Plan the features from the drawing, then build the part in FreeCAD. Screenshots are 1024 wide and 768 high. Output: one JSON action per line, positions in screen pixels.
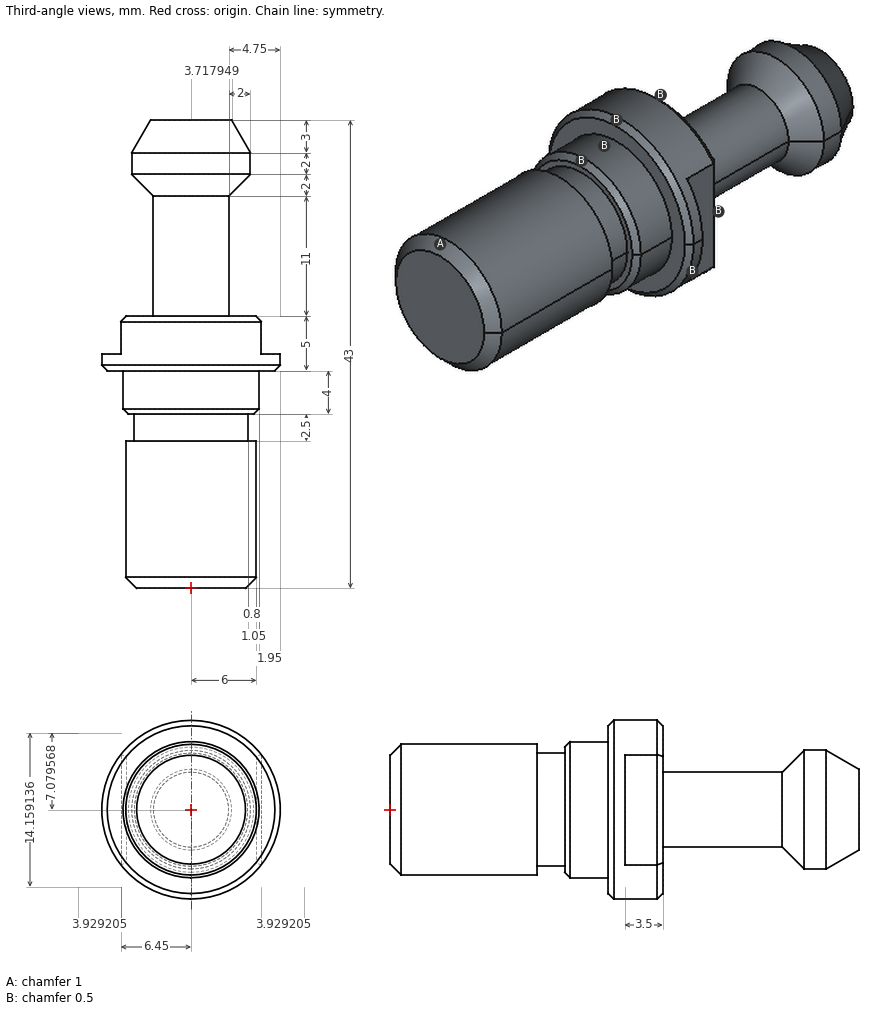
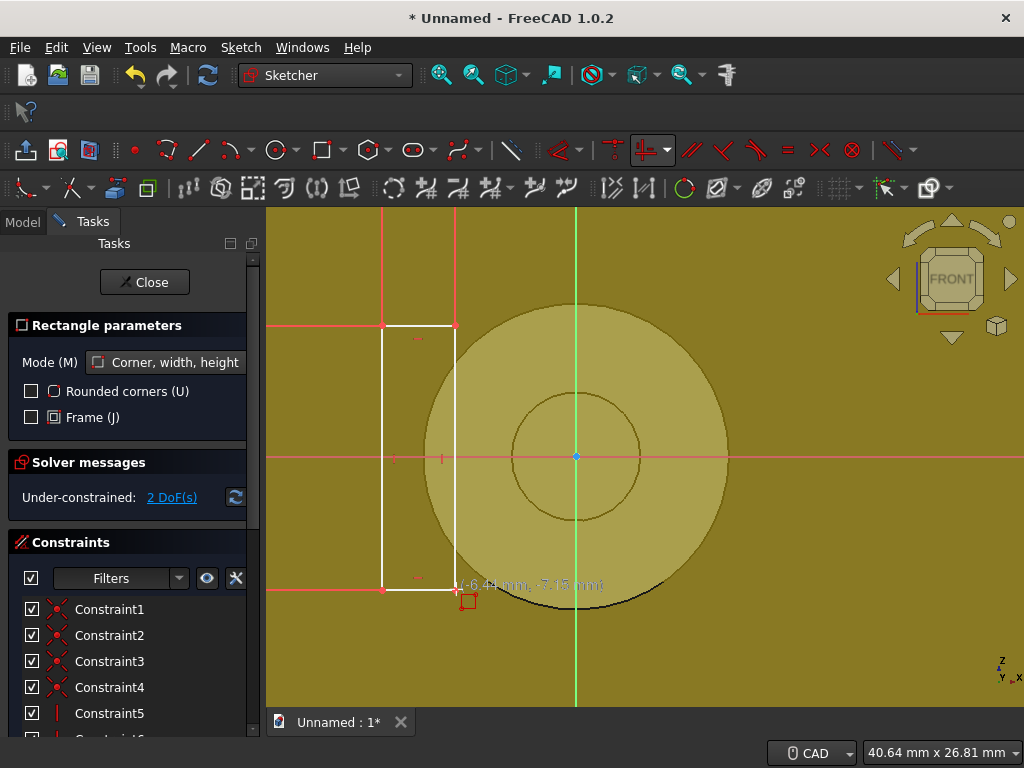
{"action": "left_click", "coordinate": [696, 325]}
{"action": "mouse_move", "coordinate": [770, 589]}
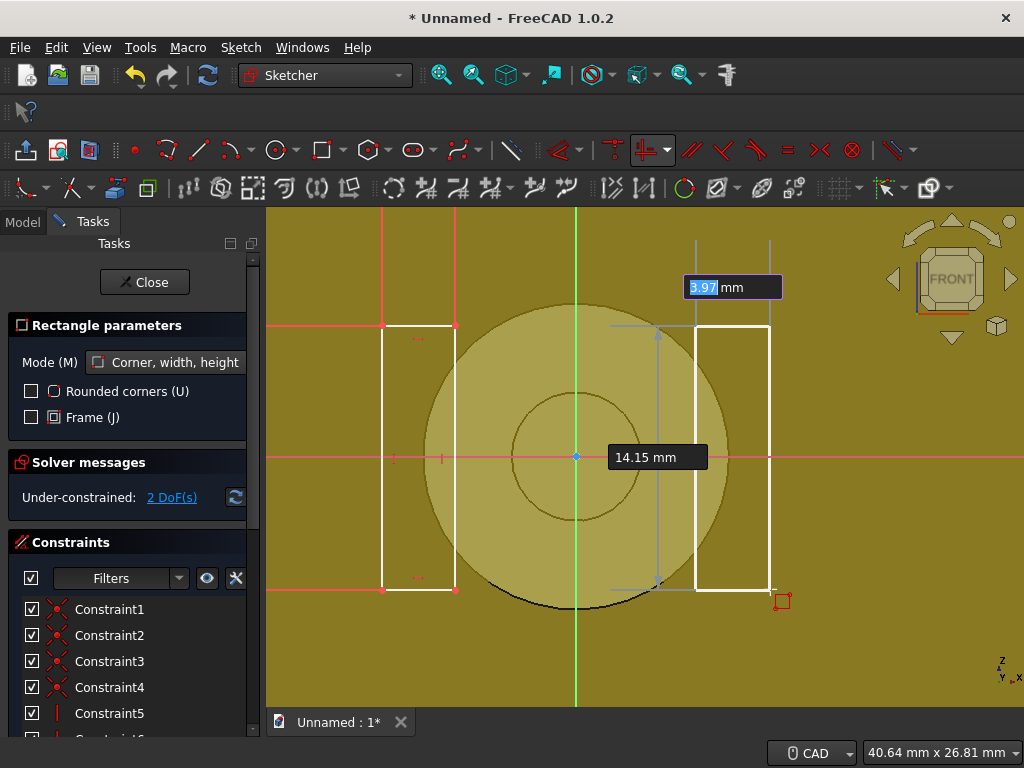
{"action": "type", "text": "3.929205"}
{"action": "key", "text": "Tab"}
{"action": "type", "text": "14.159136"}
{"action": "key", "text": "Return"}
{"action": "key", "text": "Escape"}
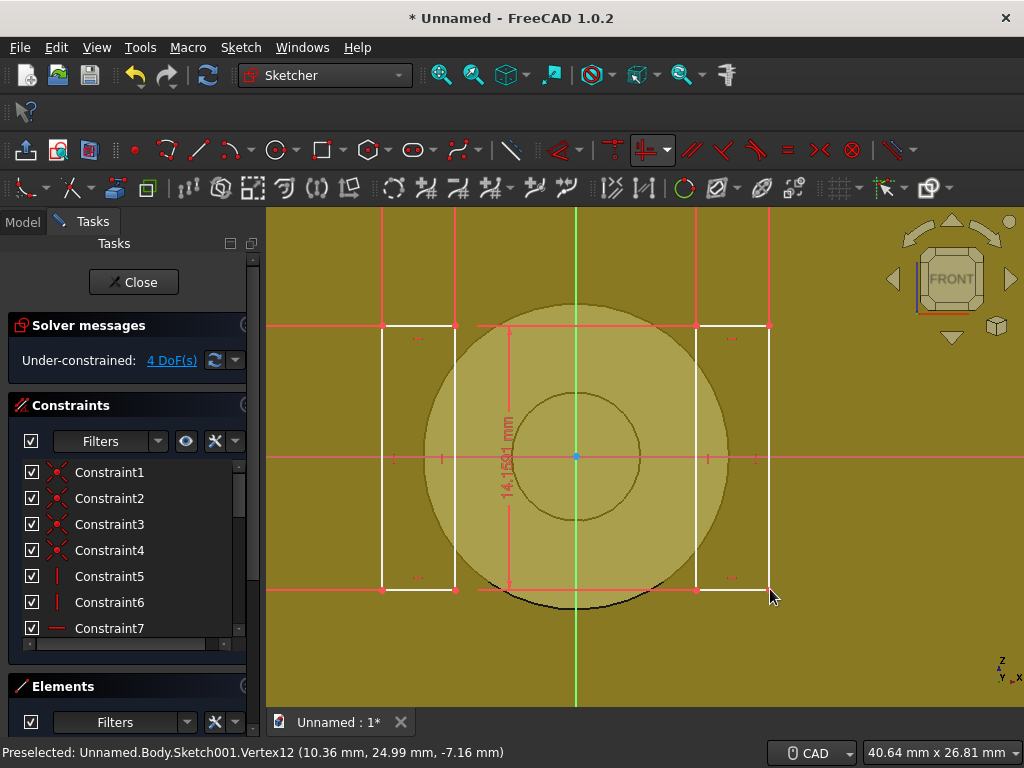
{"action": "left_click", "coordinate": [455, 326]}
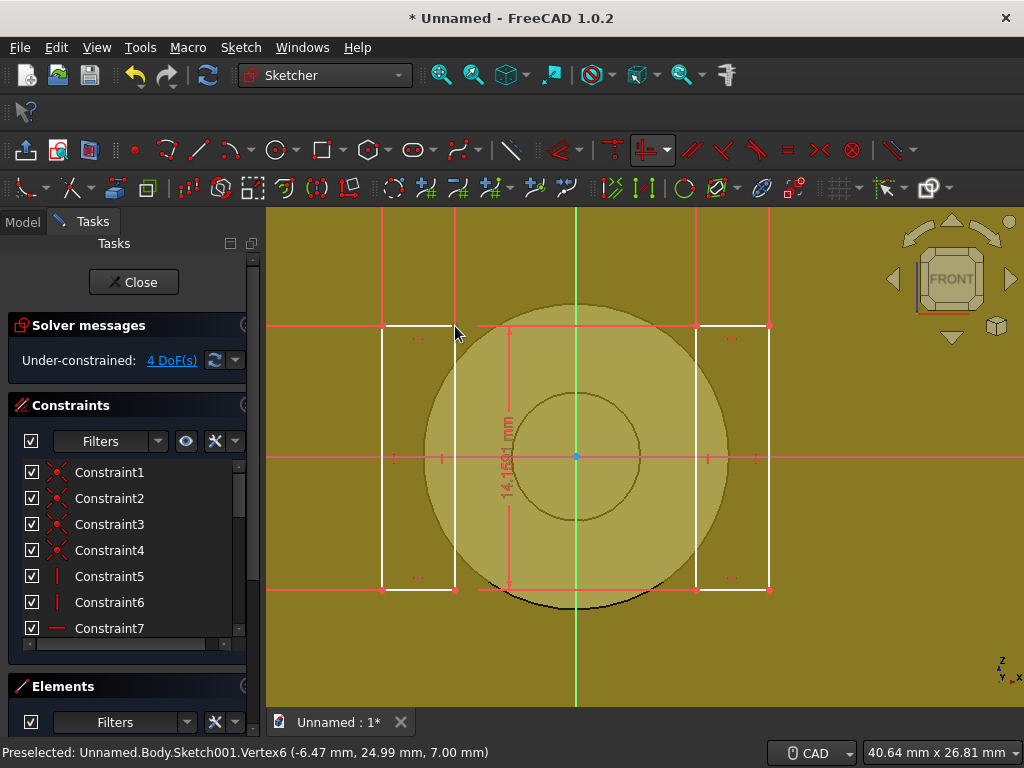
{"action": "left_click", "coordinate": [696, 326]}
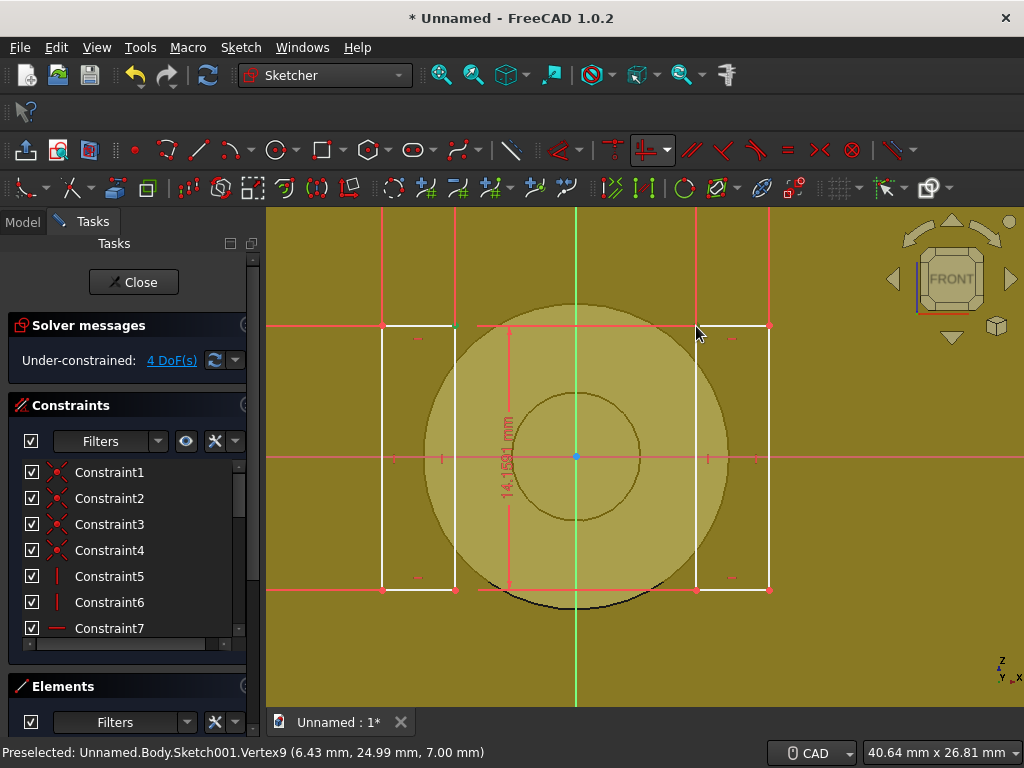
{"action": "left_click", "coordinate": [576, 647]}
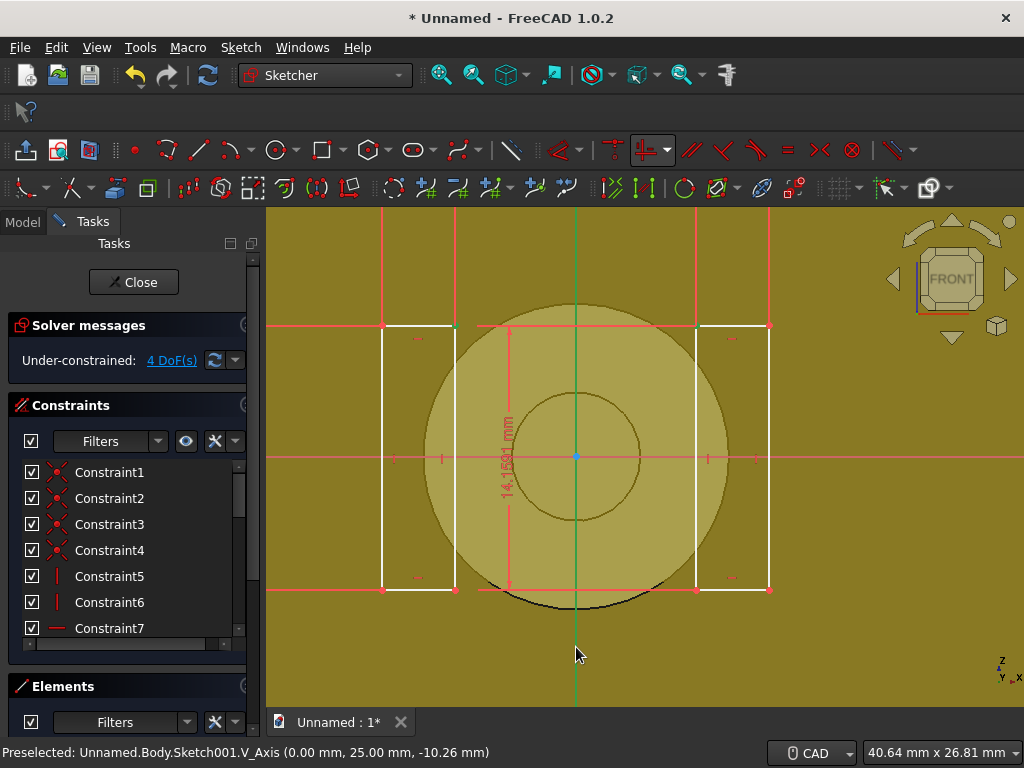
{"action": "left_click", "coordinate": [820, 150]}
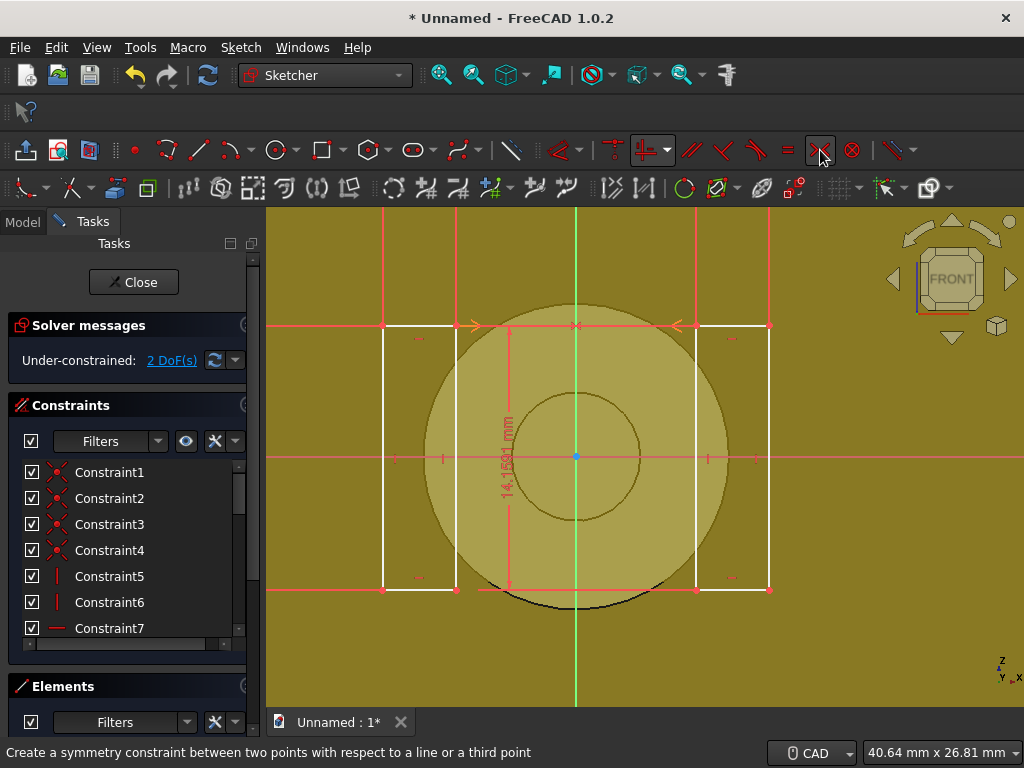
{"action": "left_click", "coordinate": [558, 150]}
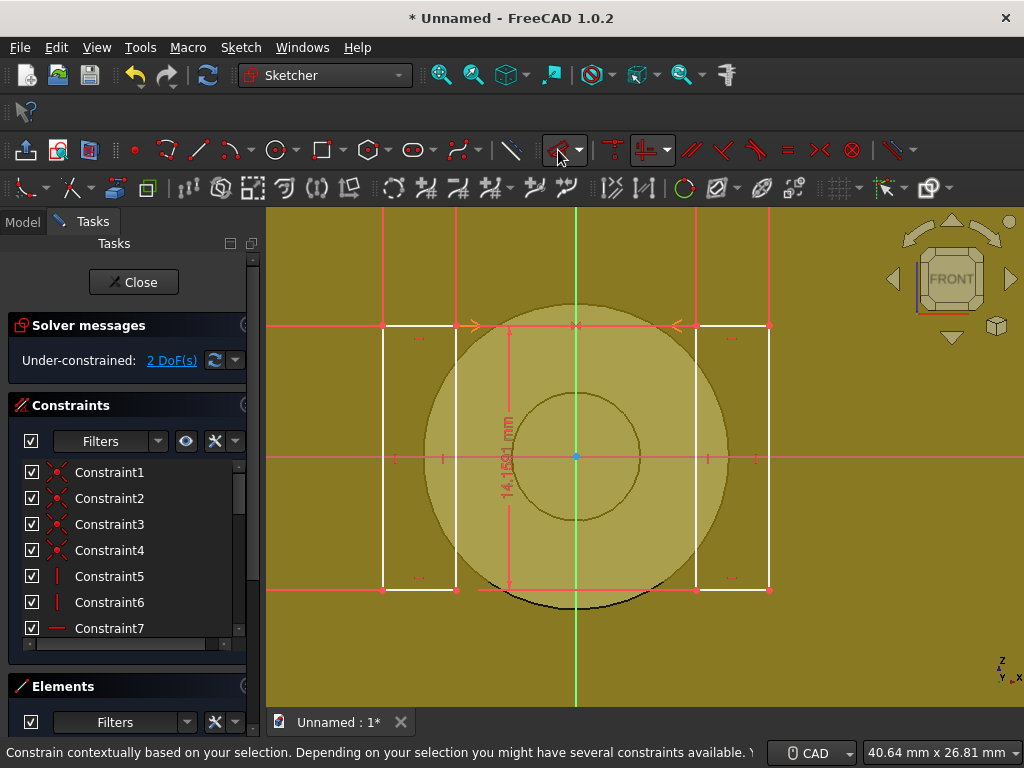
{"action": "left_click", "coordinate": [456, 590]}
{"action": "left_click", "coordinate": [516, 624]}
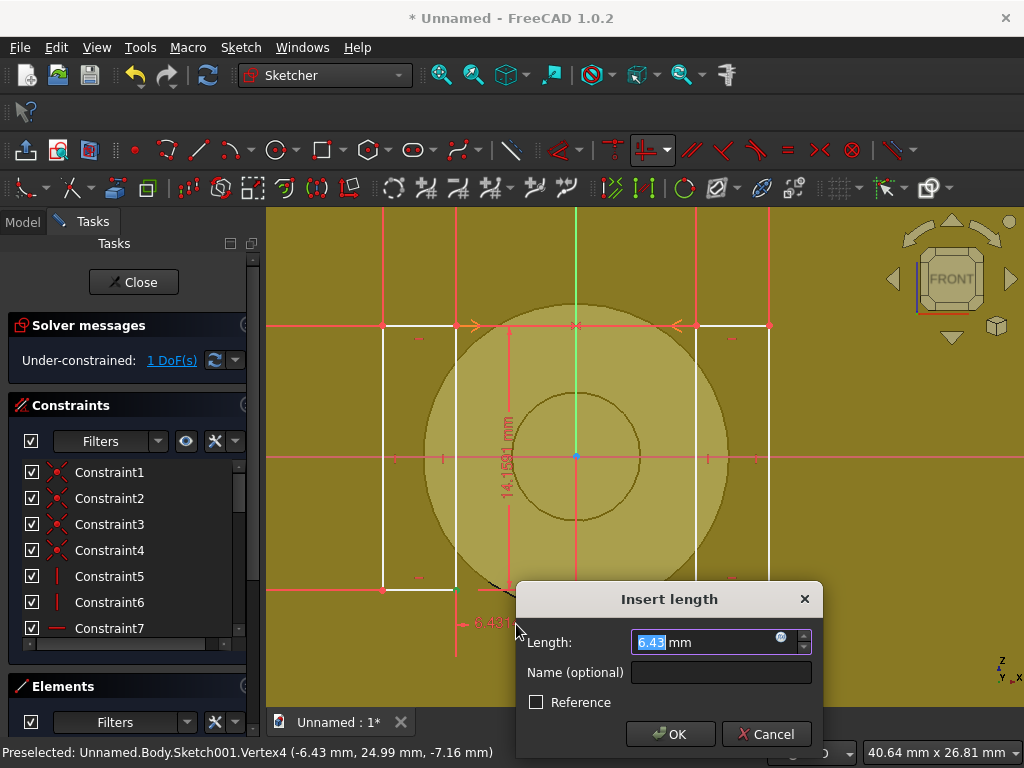
{"action": "type", "text": "6.45"}
{"action": "key", "text": "Return"}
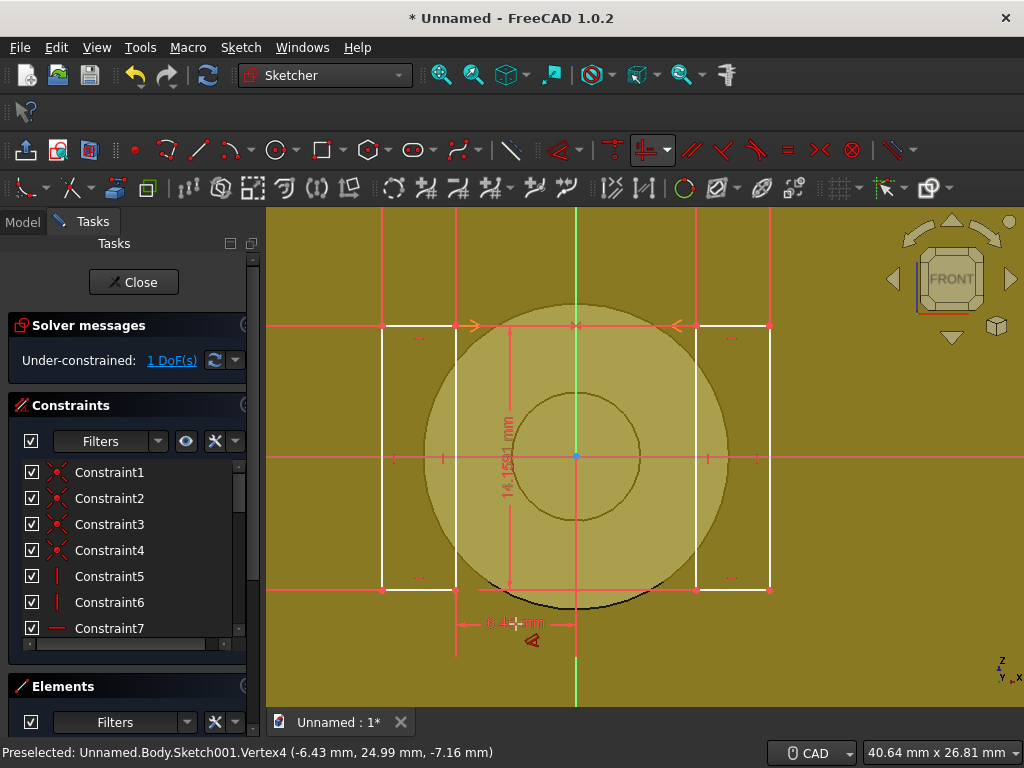
{"action": "left_click", "coordinate": [382, 326]}
{"action": "left_click", "coordinate": [348, 391]}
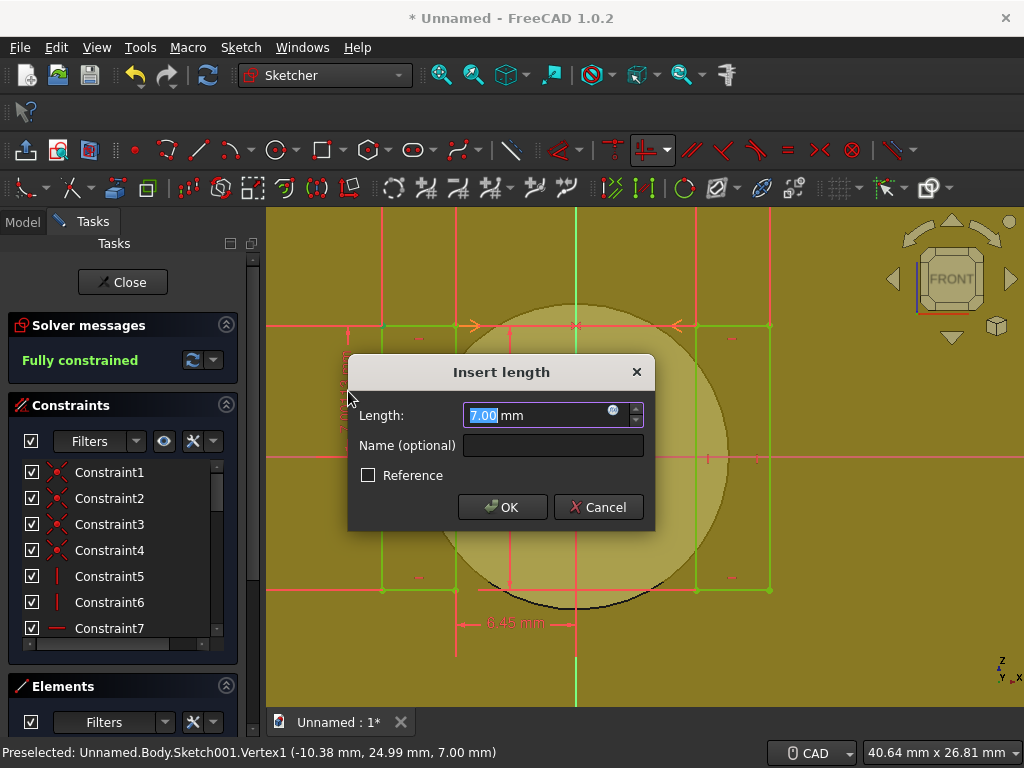
{"action": "type", "text": "7.079568"}
{"action": "key", "text": "Return"}
{"action": "key", "text": "Escape"}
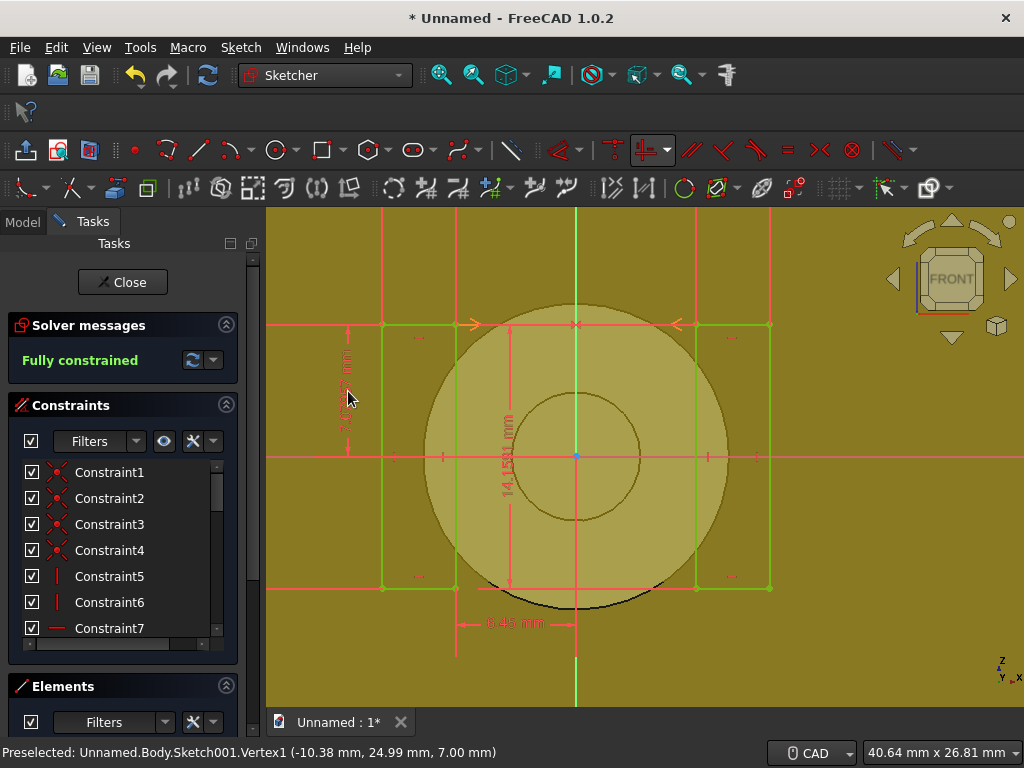
{"action": "left_click", "coordinate": [123, 282]}